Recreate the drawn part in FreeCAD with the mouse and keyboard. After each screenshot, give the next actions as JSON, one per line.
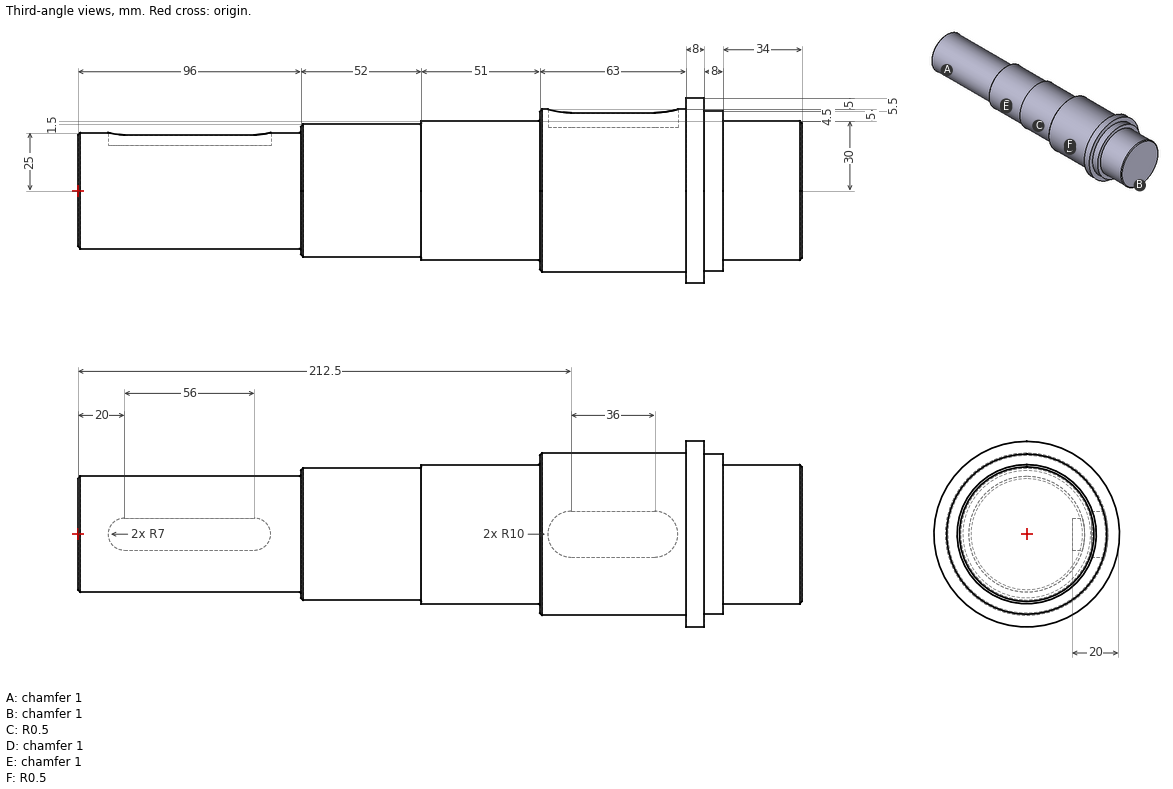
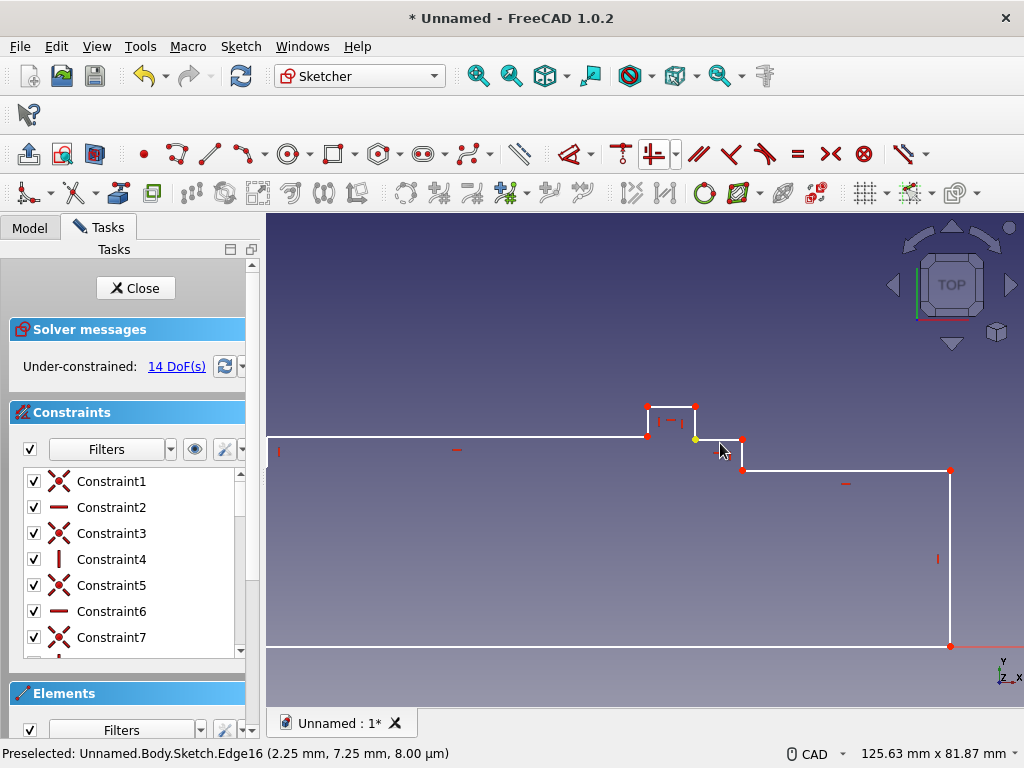
{"action": "left_click", "coordinate": [719, 440]}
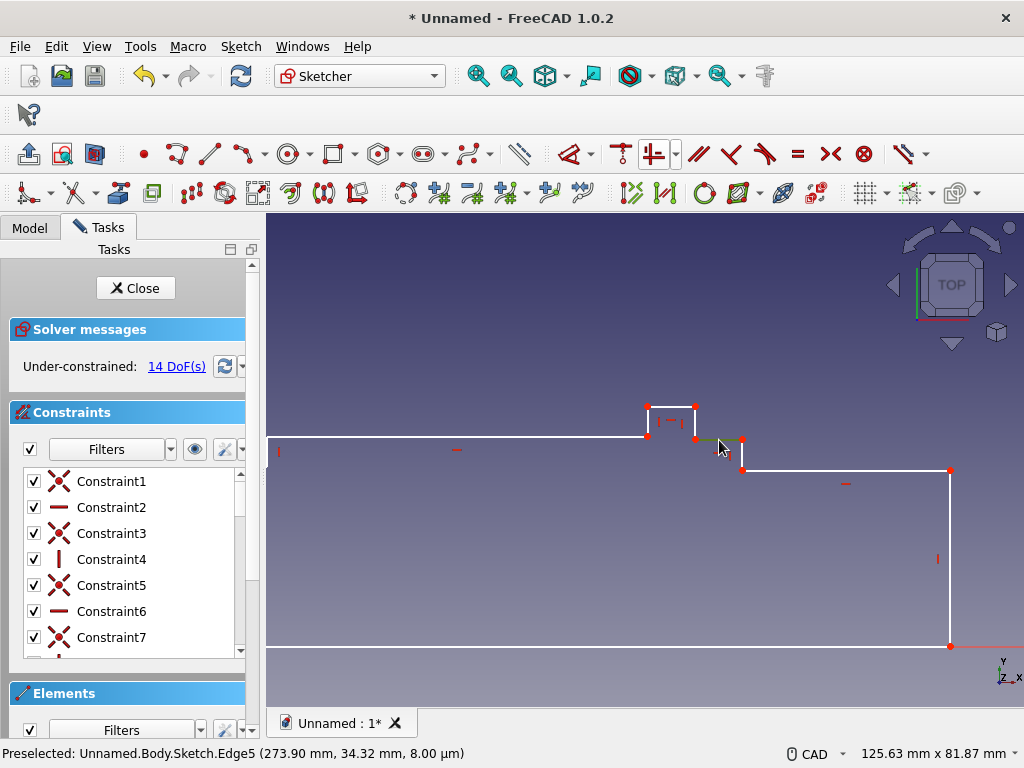
{"action": "key", "text": "l"}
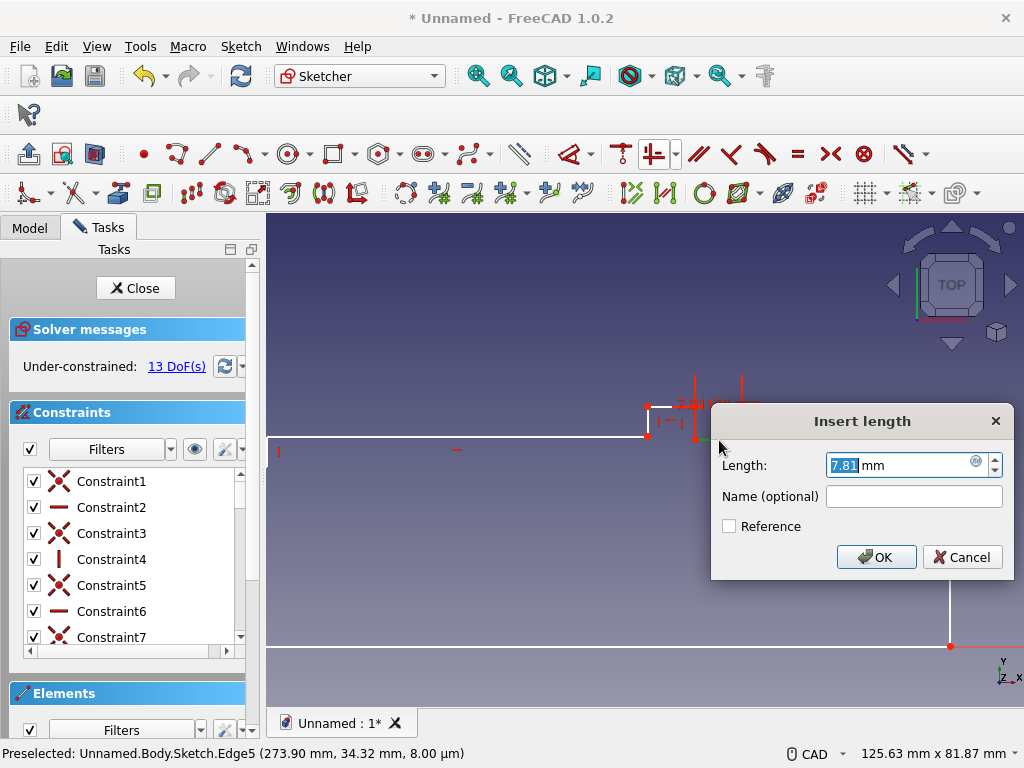
{"action": "type", "text": "8"}
{"action": "key", "text": "Return"}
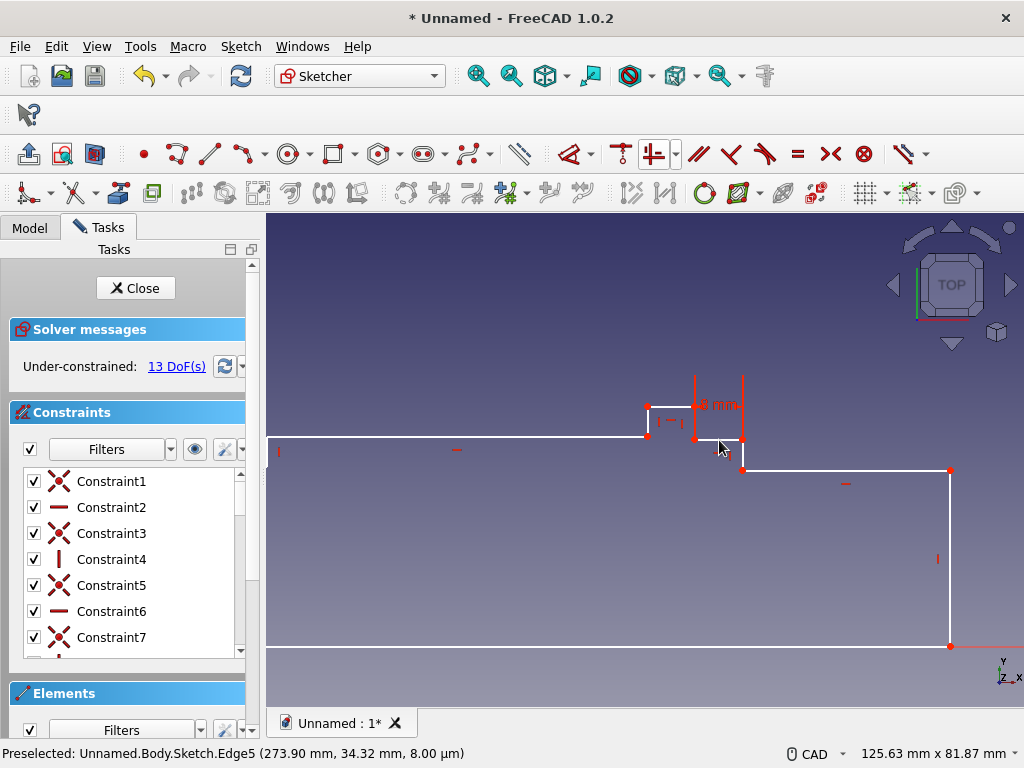
{"action": "left_click", "coordinate": [680, 407]}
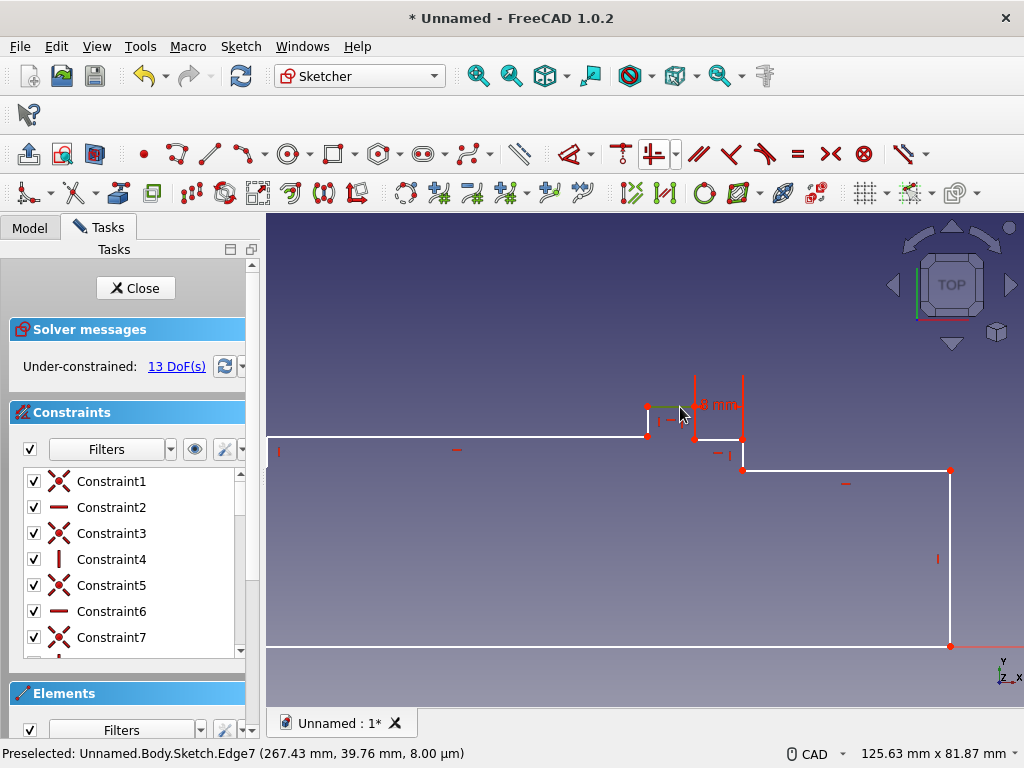
{"action": "left_click", "coordinate": [590, 154]}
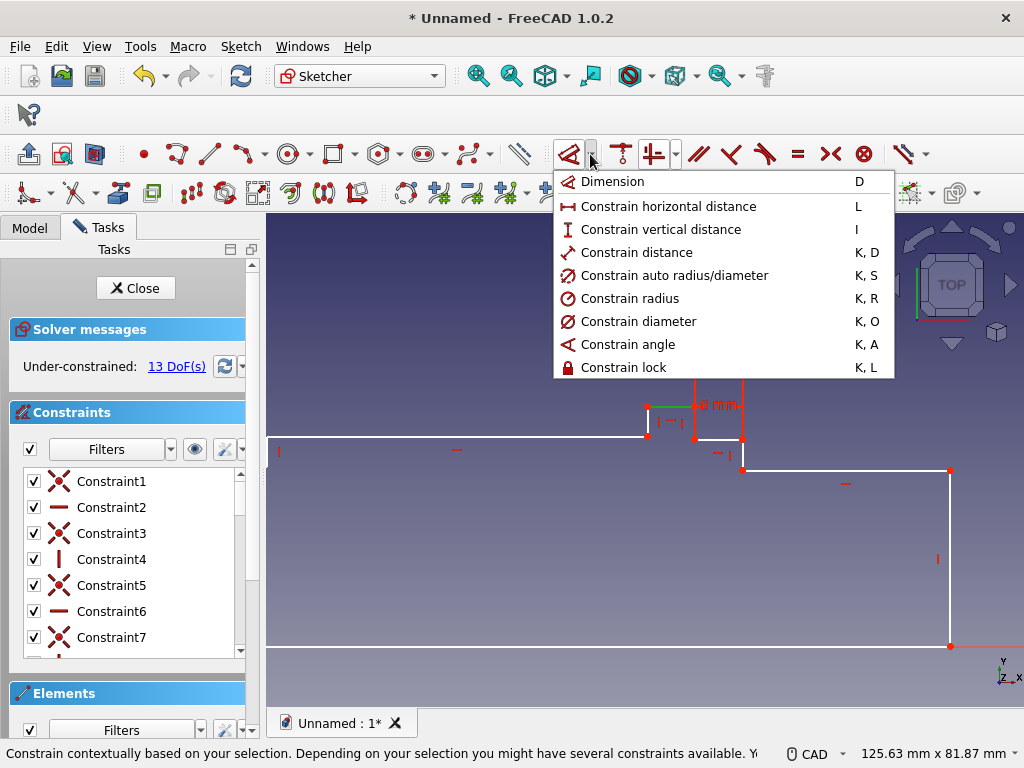
{"action": "left_click", "coordinate": [724, 206]}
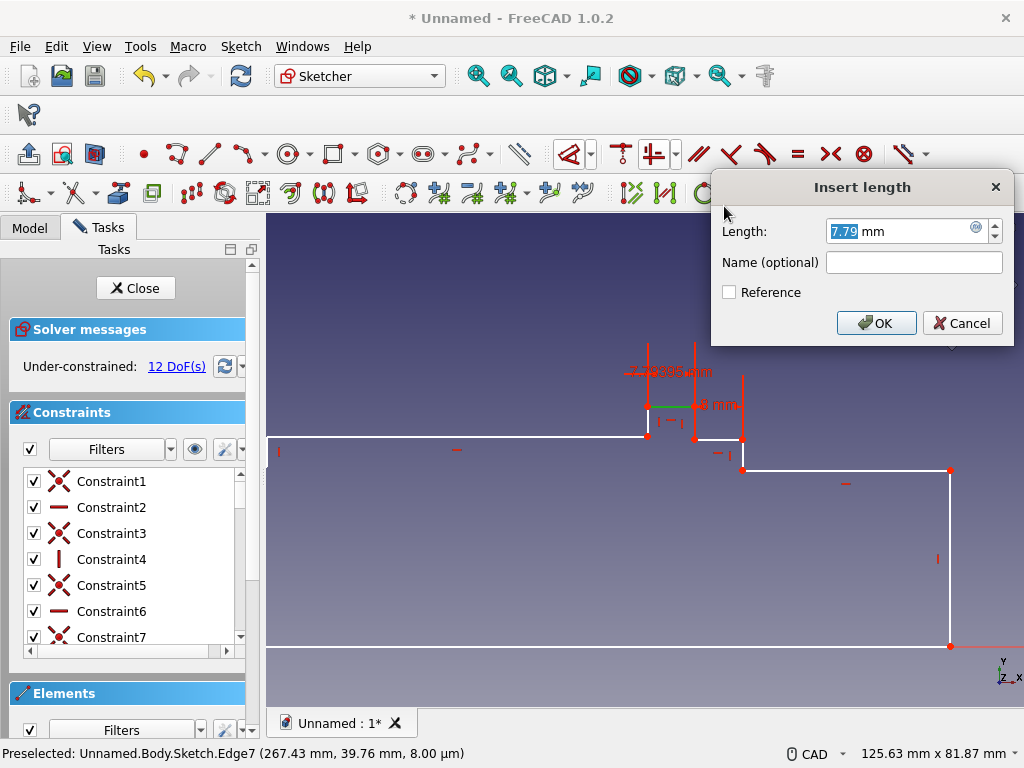
{"action": "type", "text": "8"}
{"action": "key", "text": "Return"}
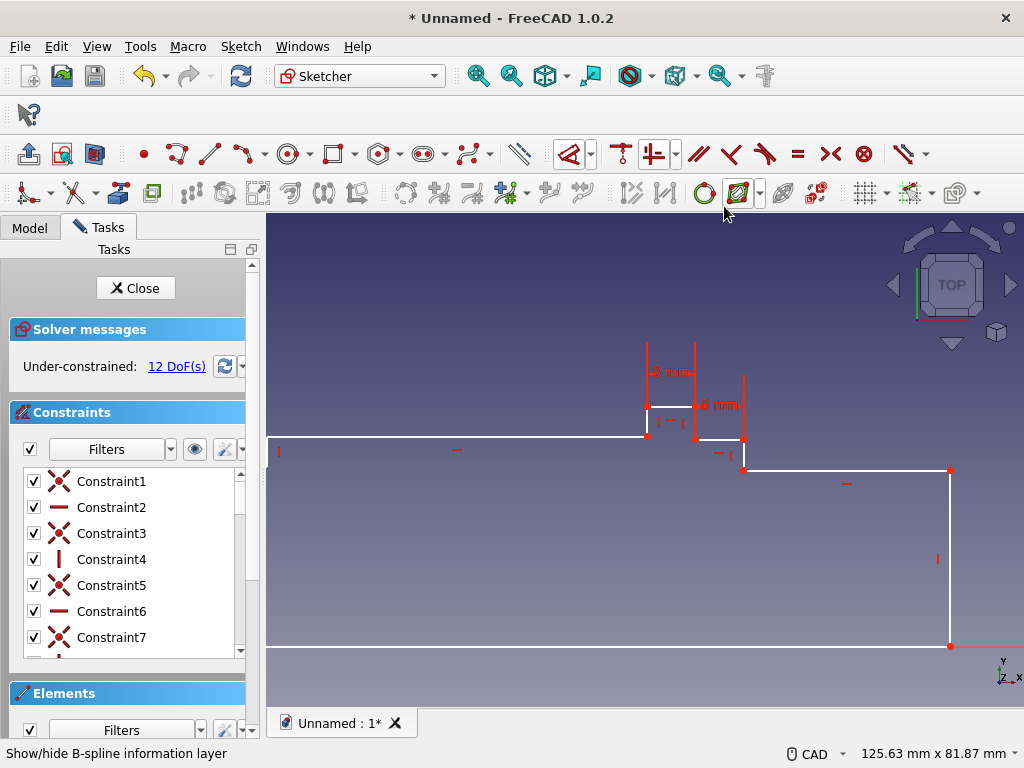
{"action": "scroll", "coordinate": [647, 419], "scroll_direction": "up", "scroll_amount": 2}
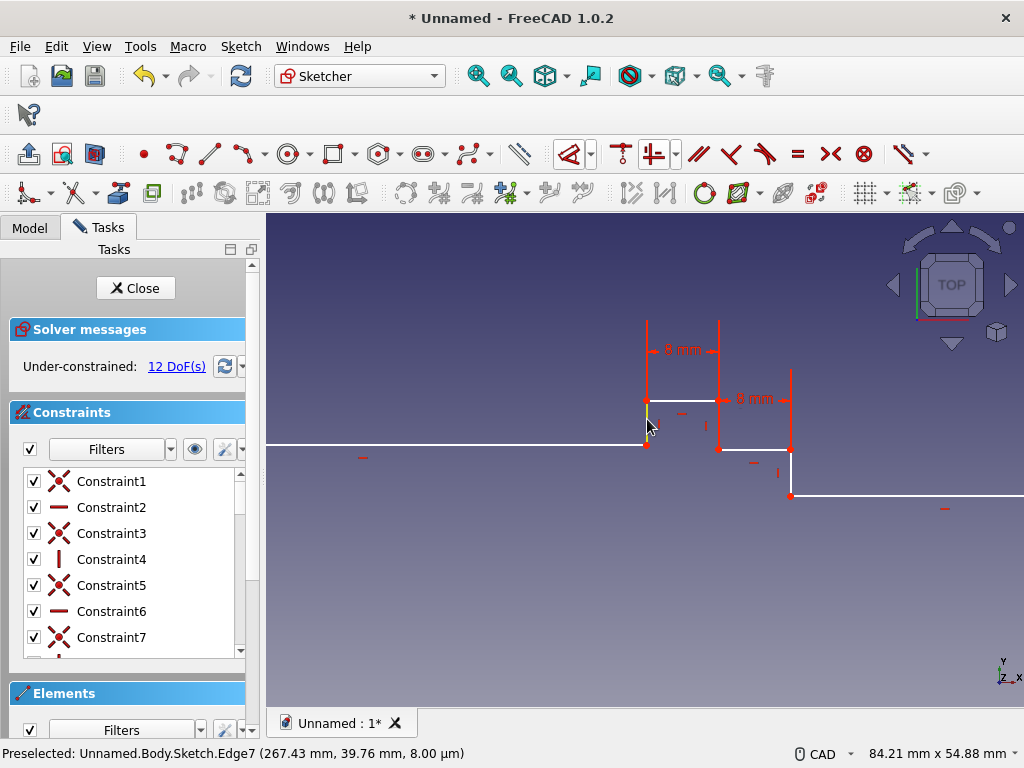
{"action": "left_click", "coordinate": [647, 419]}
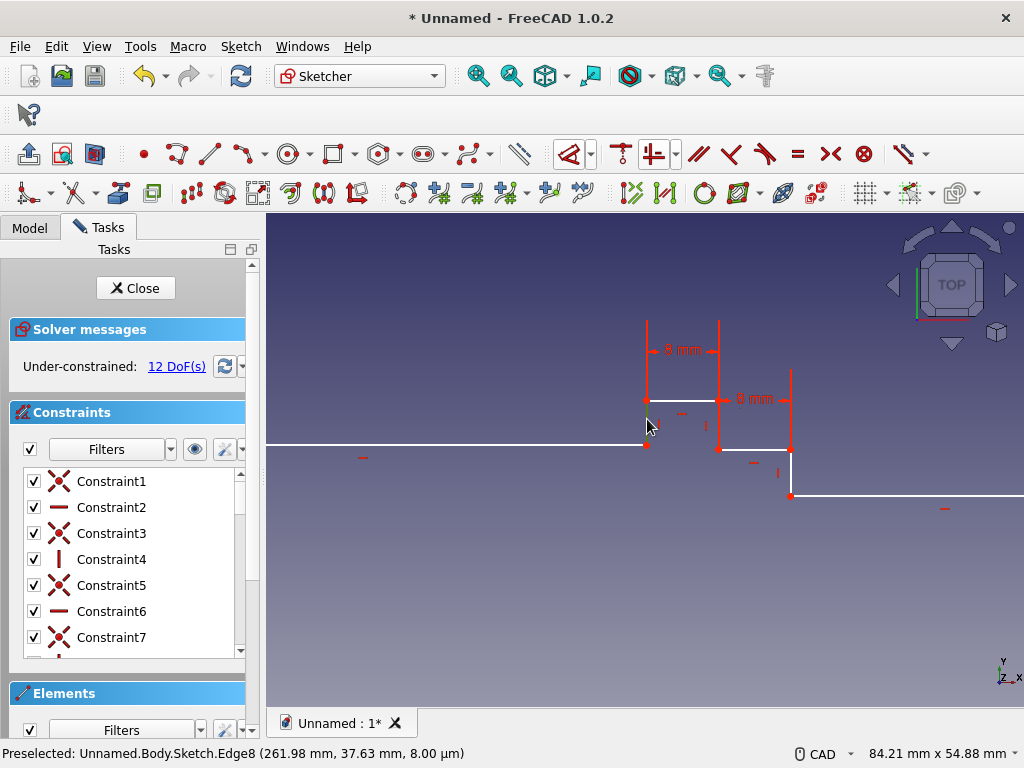
{"action": "left_click", "coordinate": [590, 154]}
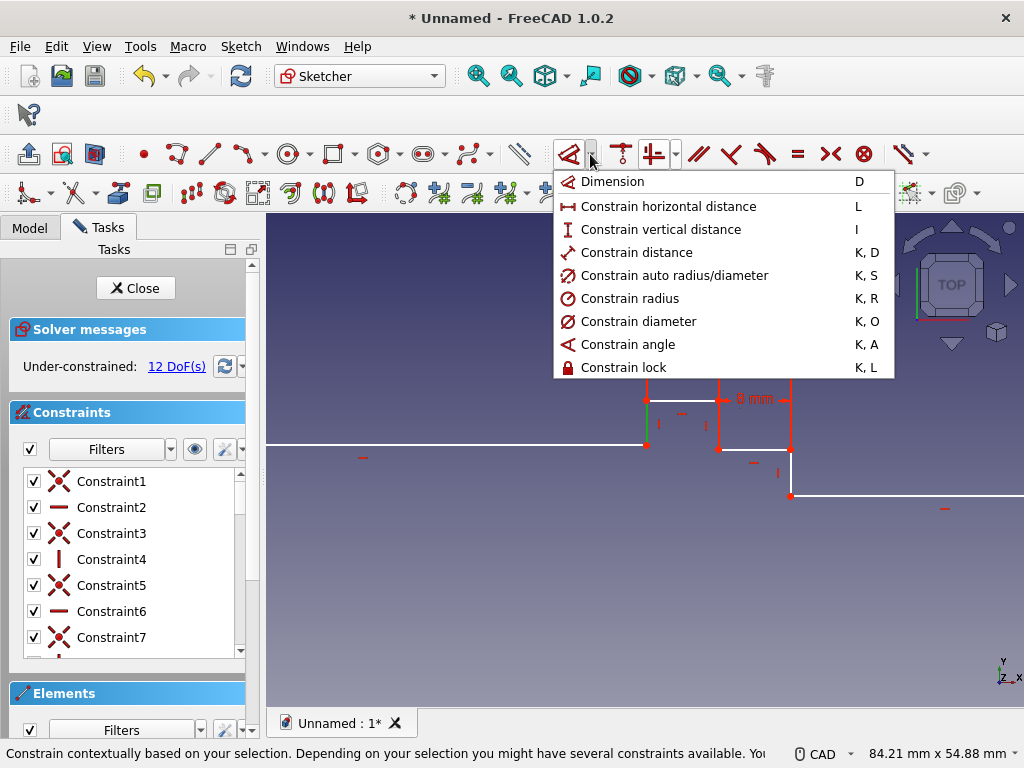
{"action": "left_click", "coordinate": [724, 230]}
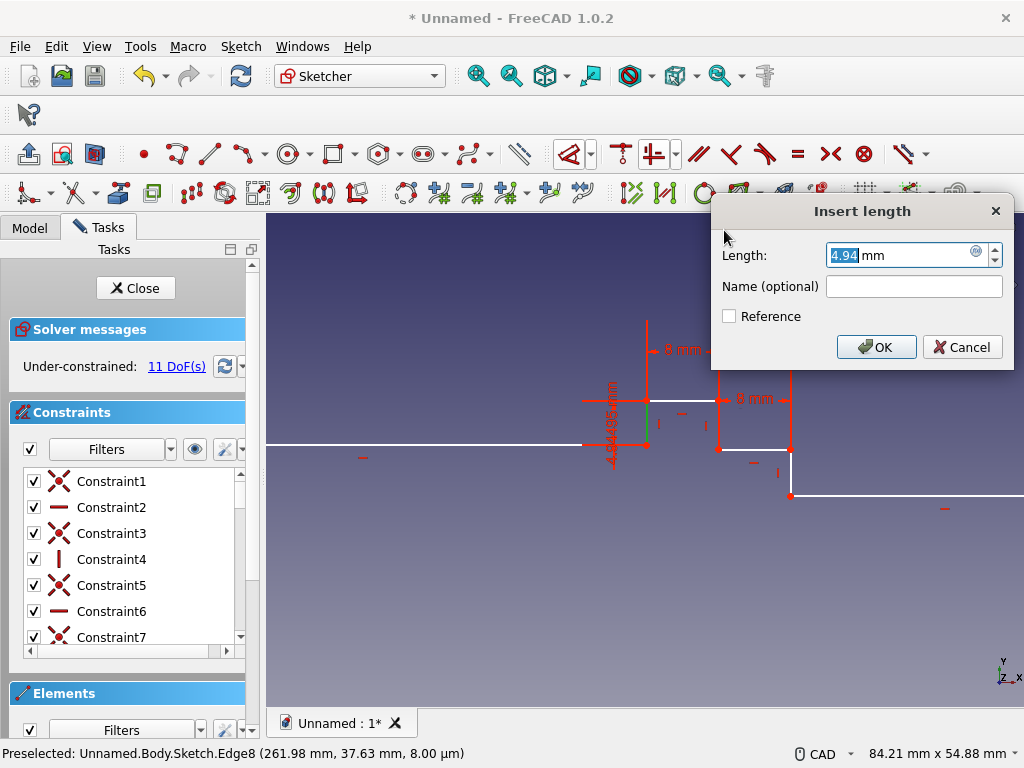
{"action": "type", "text": "5"}
{"action": "key", "text": "Return"}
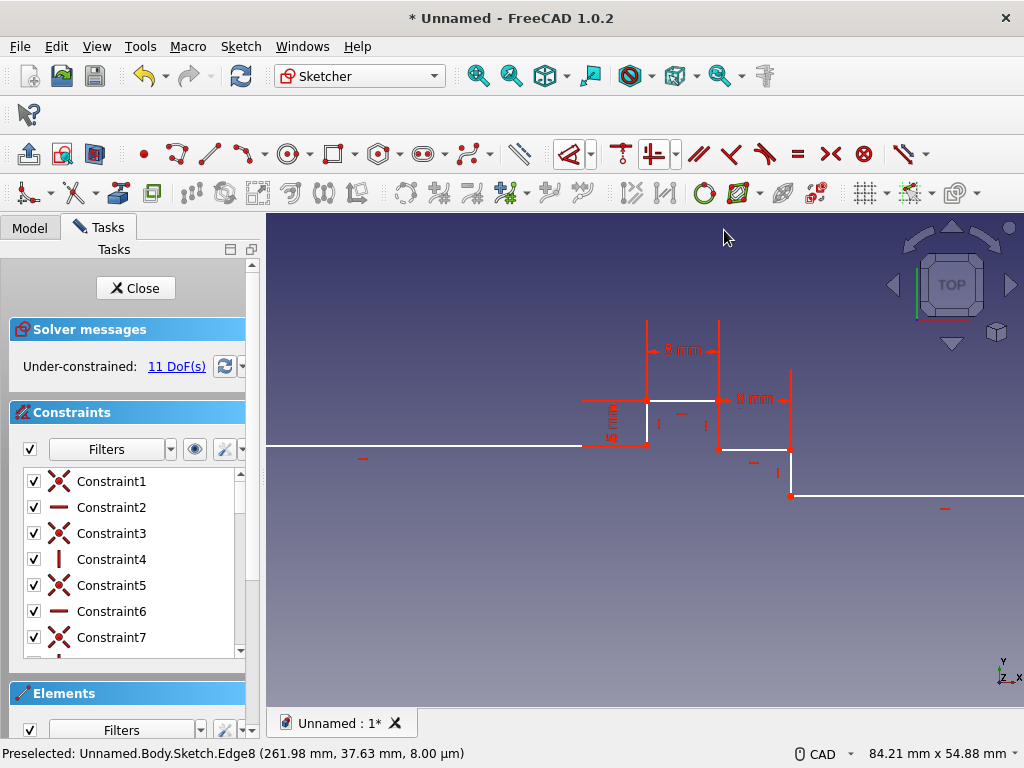
{"action": "scroll", "coordinate": [715, 441], "scroll_direction": "down", "scroll_amount": 10}